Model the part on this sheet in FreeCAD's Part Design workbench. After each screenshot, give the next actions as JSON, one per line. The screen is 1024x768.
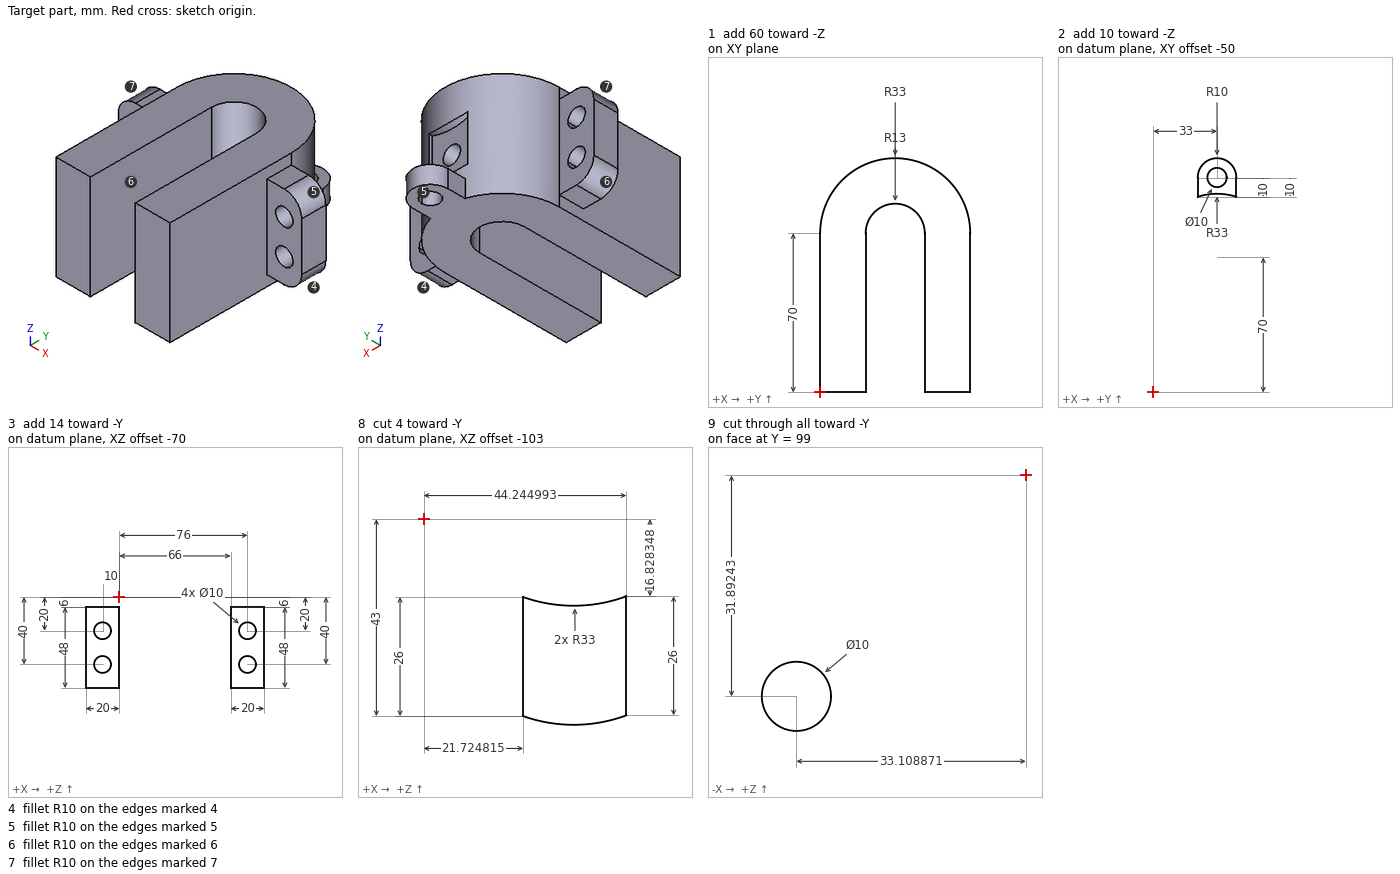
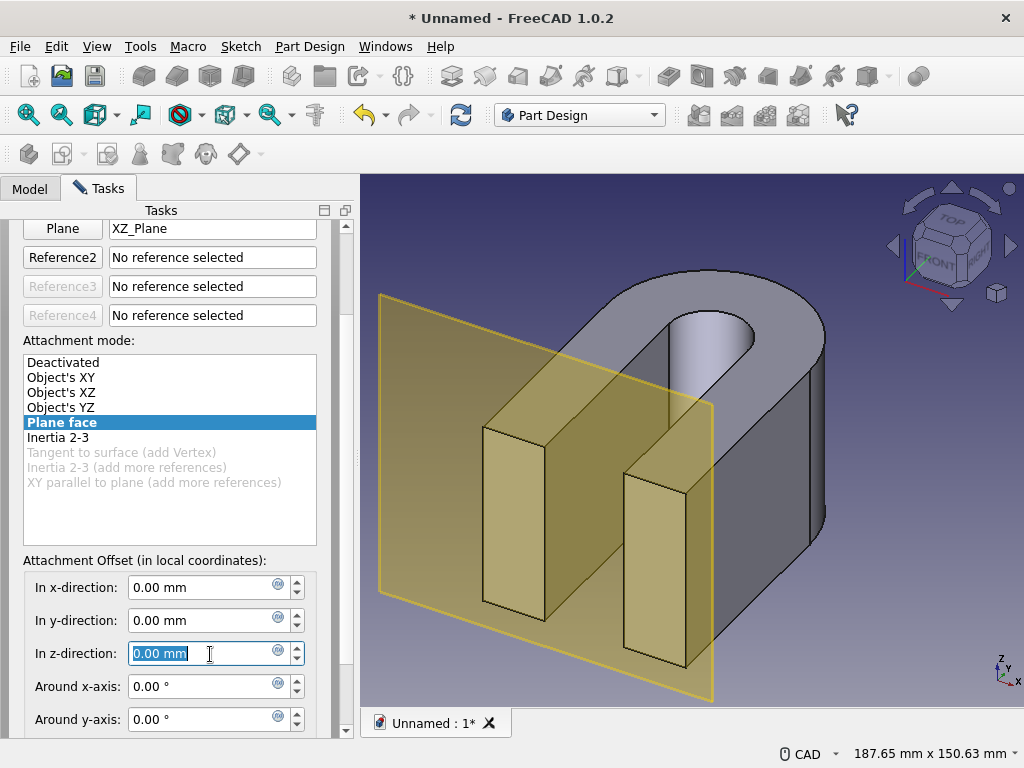
{"action": "type", "text": "-70"}
{"action": "key", "text": "Tab"}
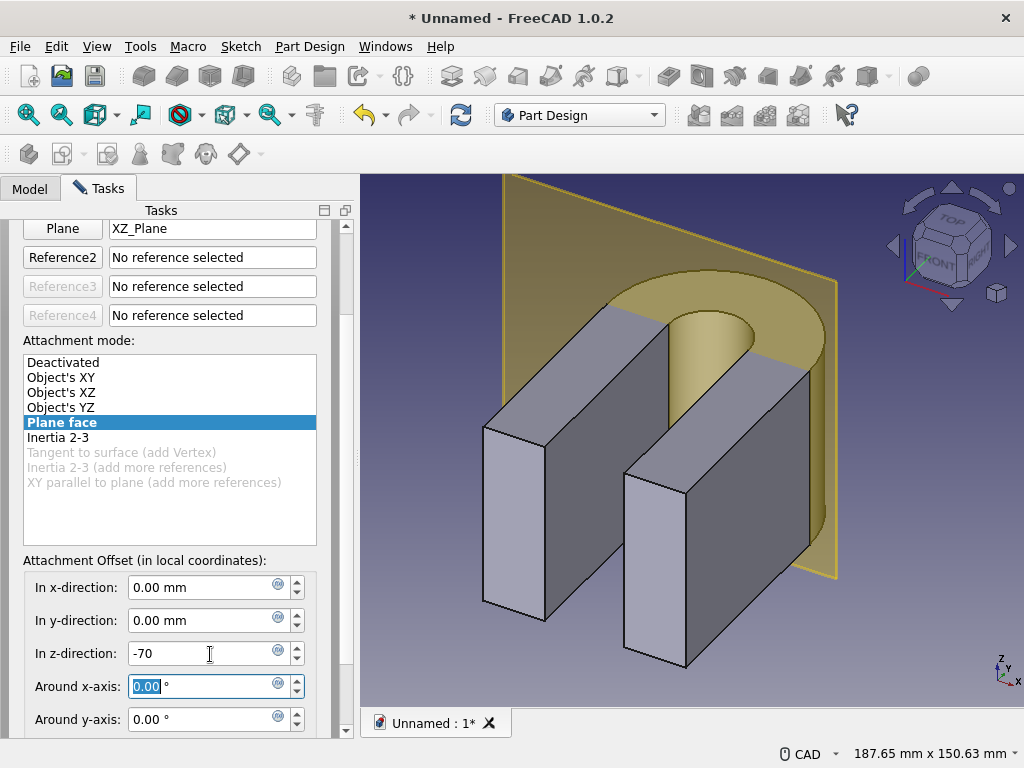
{"action": "scroll", "coordinate": [346, 479], "scroll_direction": "up", "scroll_amount": 3}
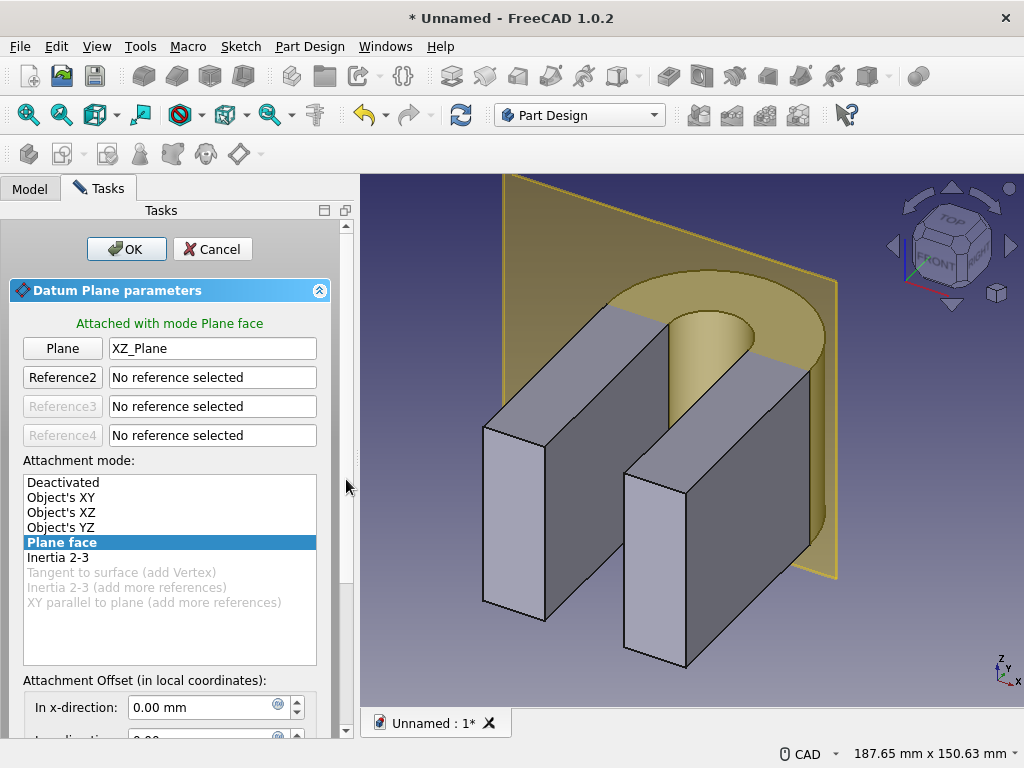
{"action": "left_click", "coordinate": [127, 249]}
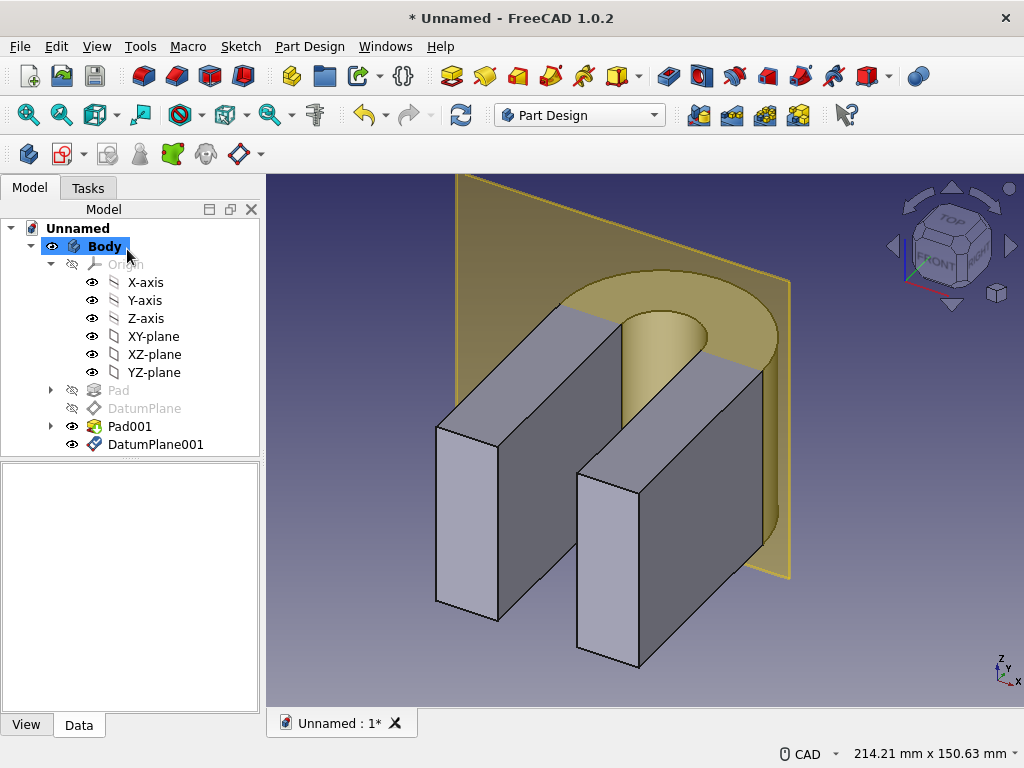
{"action": "left_click", "coordinate": [117, 444]}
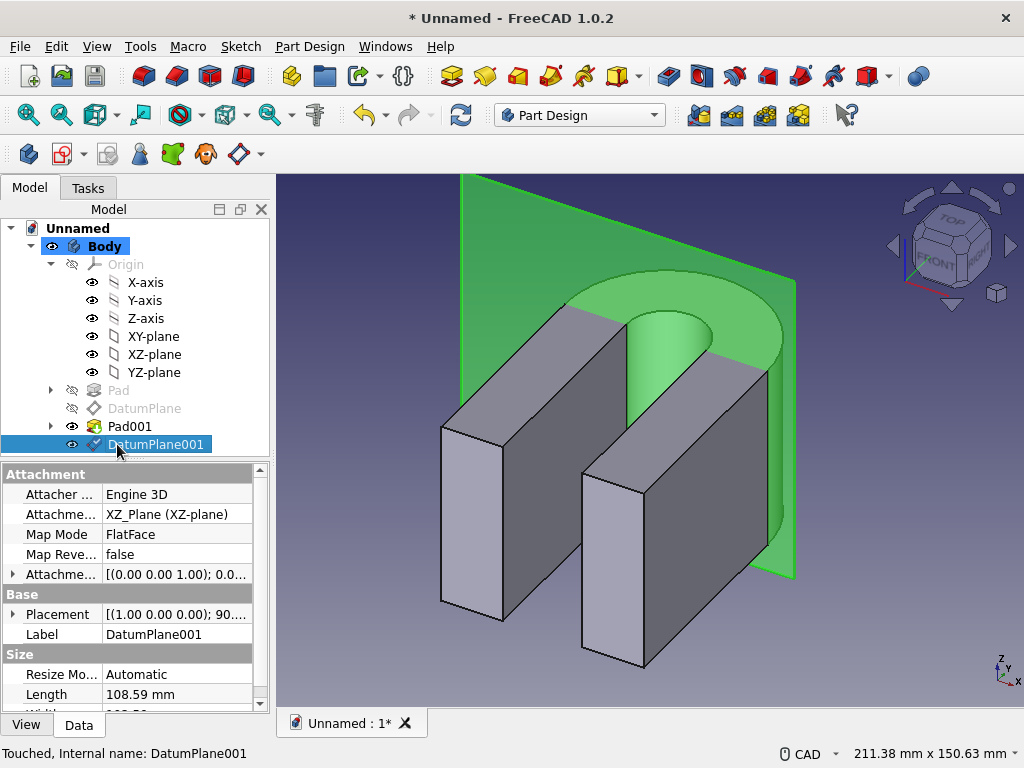
{"action": "left_click", "coordinate": [62, 154]}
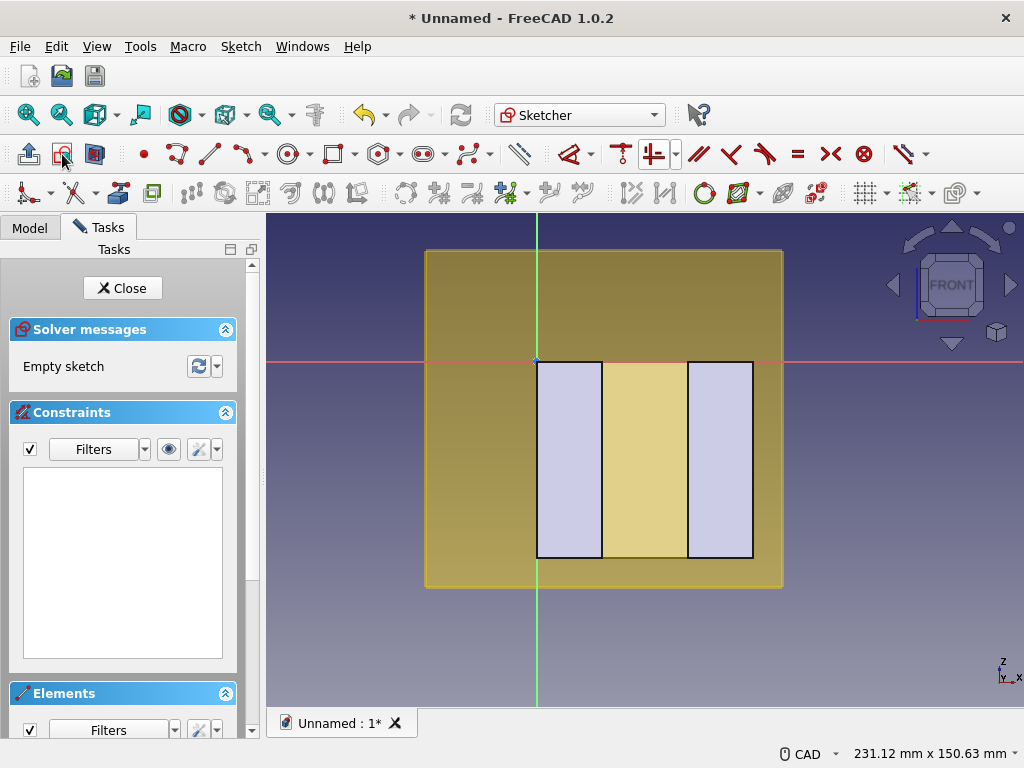
{"action": "left_click", "coordinate": [95, 154]}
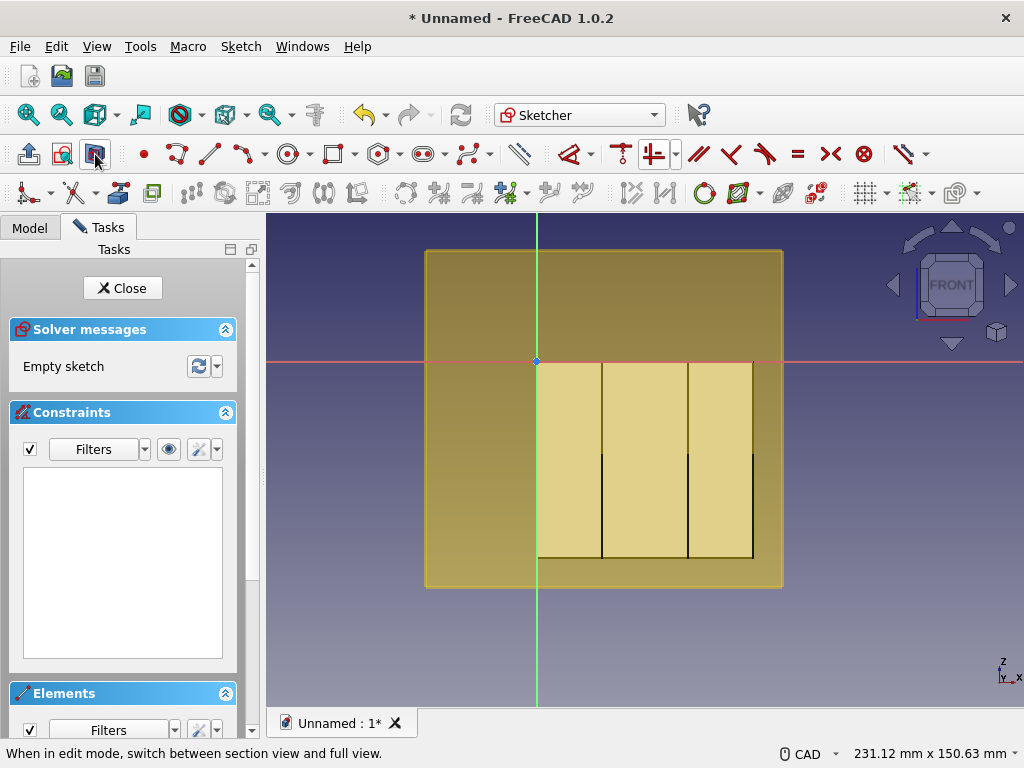
{"action": "left_click", "coordinate": [332, 154]}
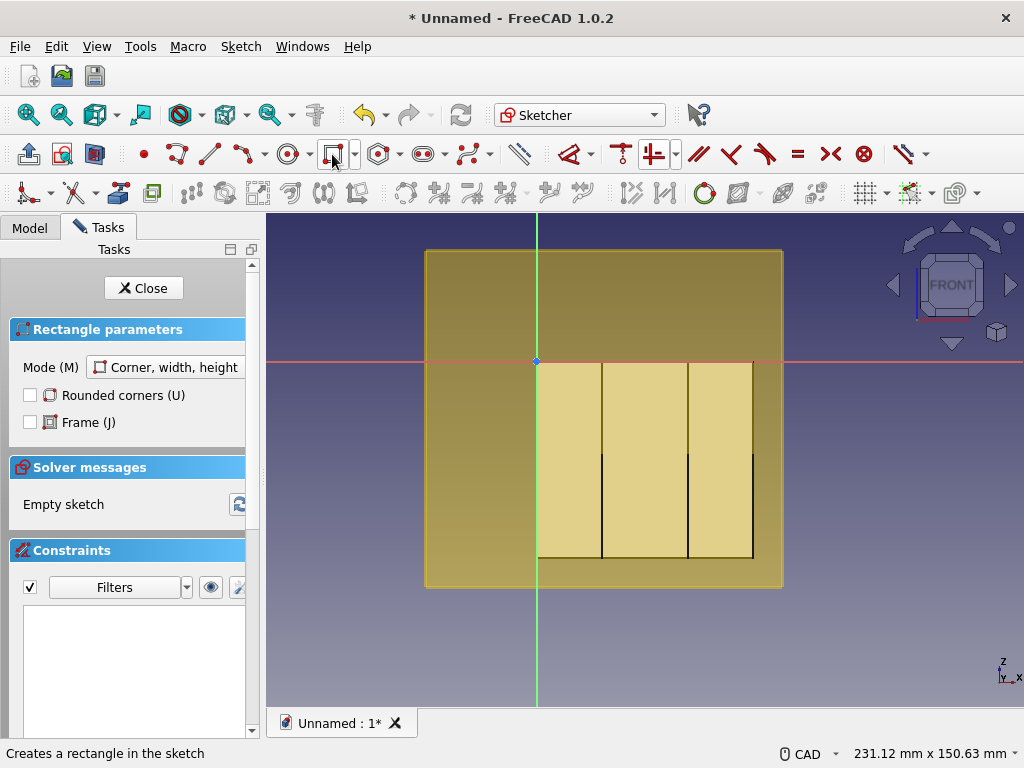
{"action": "left_click", "coordinate": [753, 381]}
{"action": "mouse_move", "coordinate": [819, 539]}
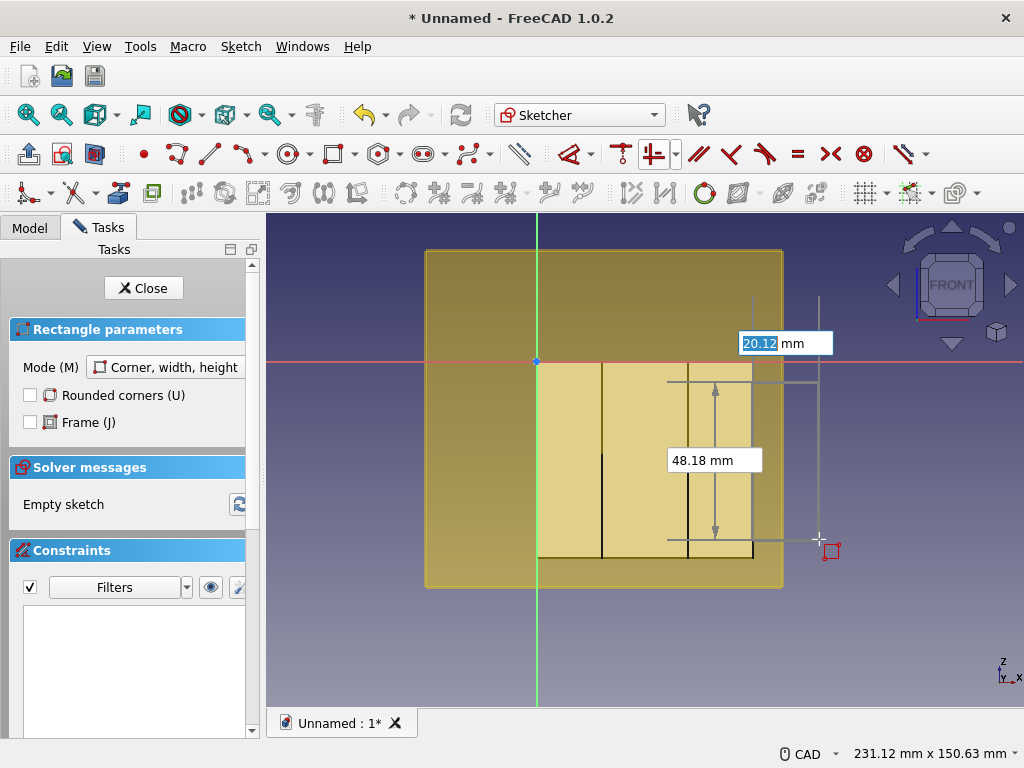
{"action": "type", "text": "20"}
{"action": "key", "text": "Tab"}
{"action": "type", "text": "48"}
{"action": "key", "text": "Return"}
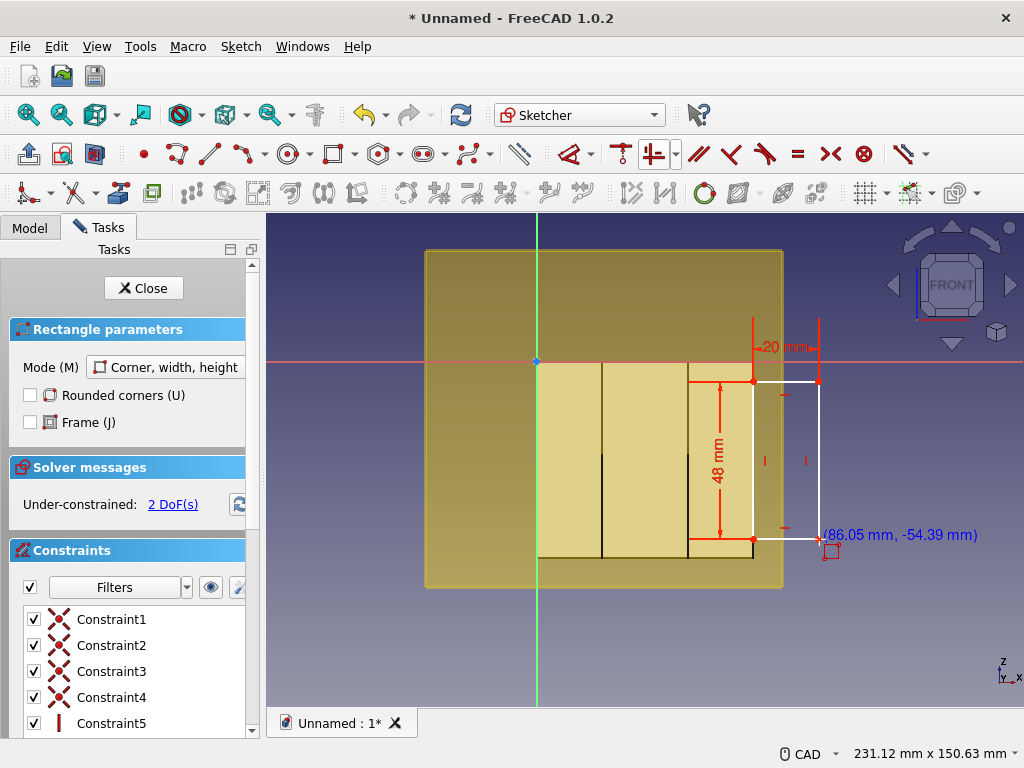
{"action": "left_click", "coordinate": [471, 381]}
{"action": "left_click", "coordinate": [537, 539]}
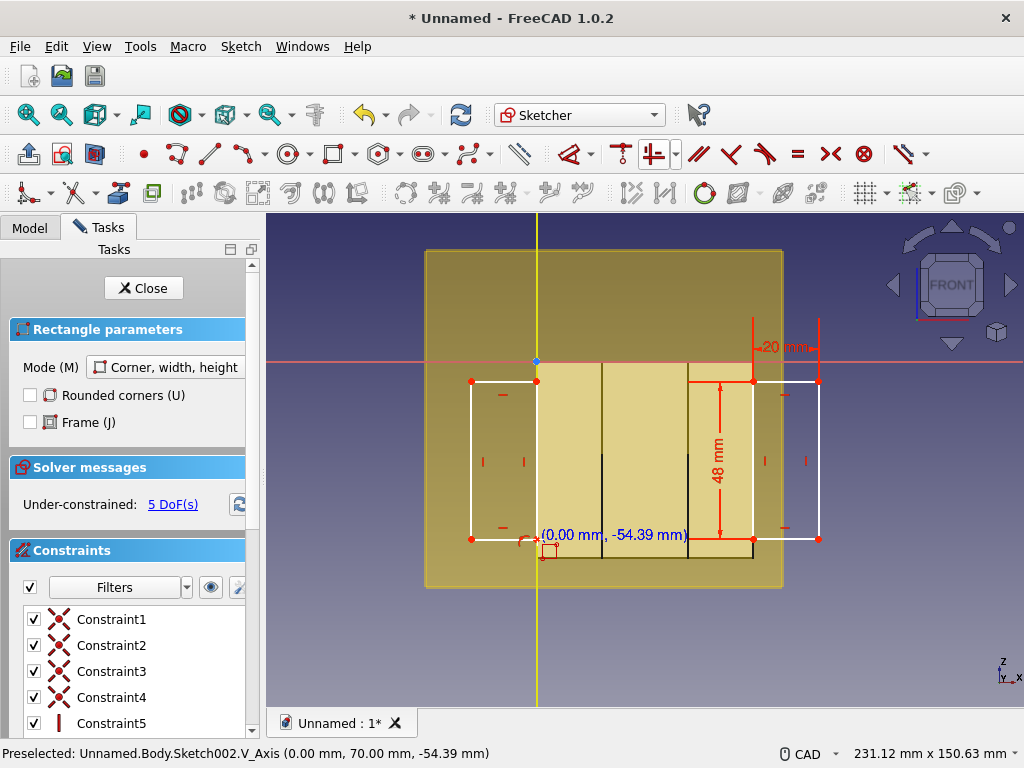
{"action": "key", "text": "g c"}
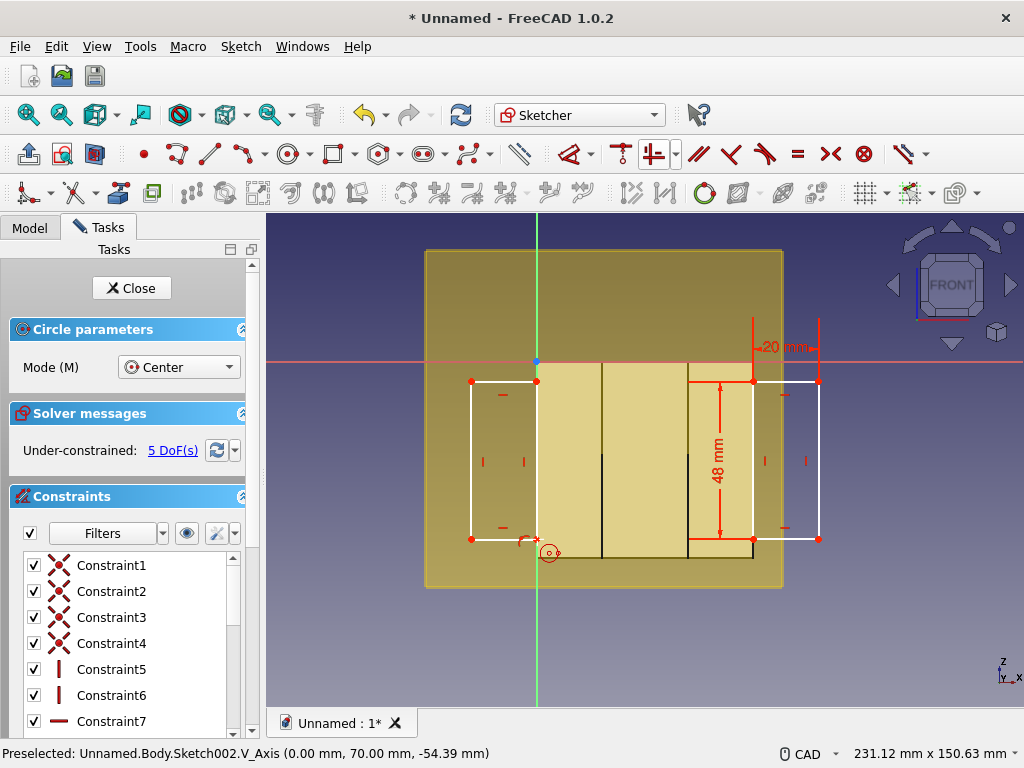
{"action": "scroll", "coordinate": [786, 427], "scroll_direction": "up", "scroll_amount": 2}